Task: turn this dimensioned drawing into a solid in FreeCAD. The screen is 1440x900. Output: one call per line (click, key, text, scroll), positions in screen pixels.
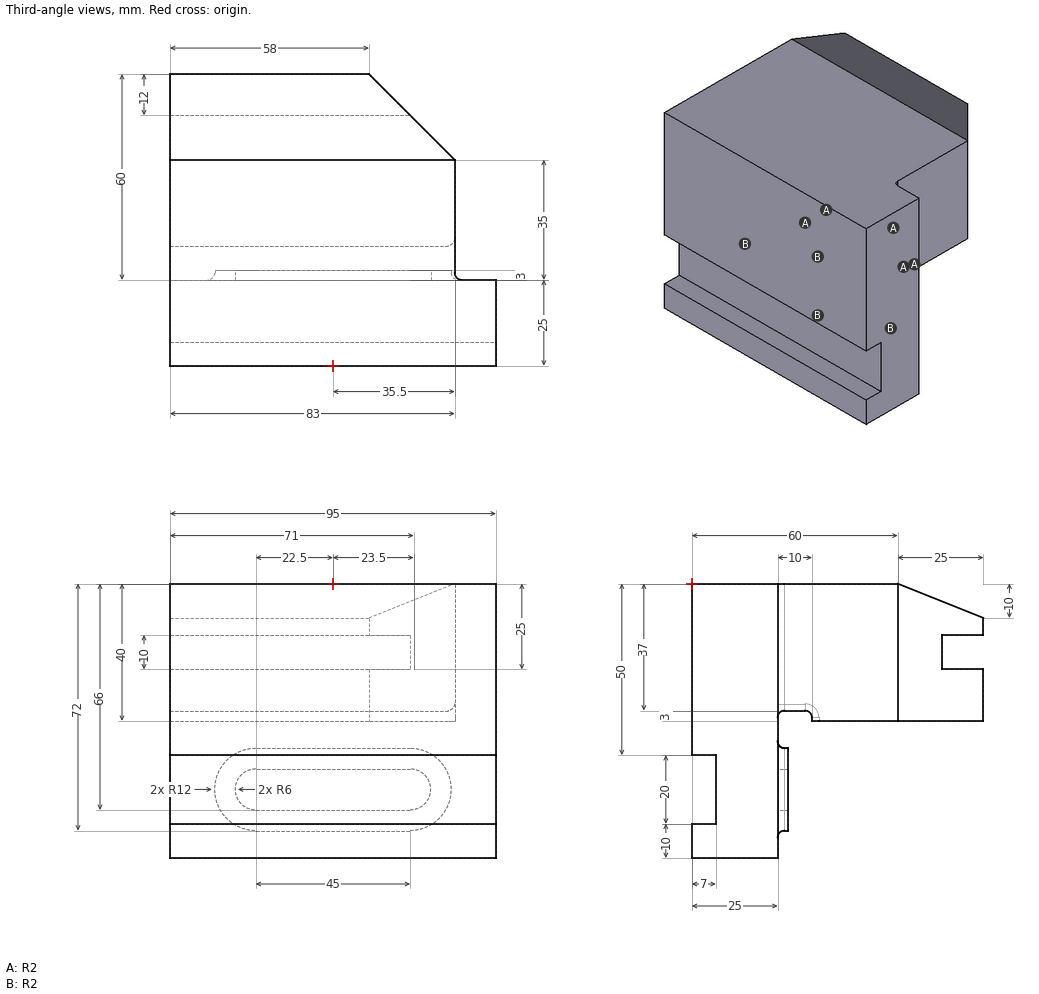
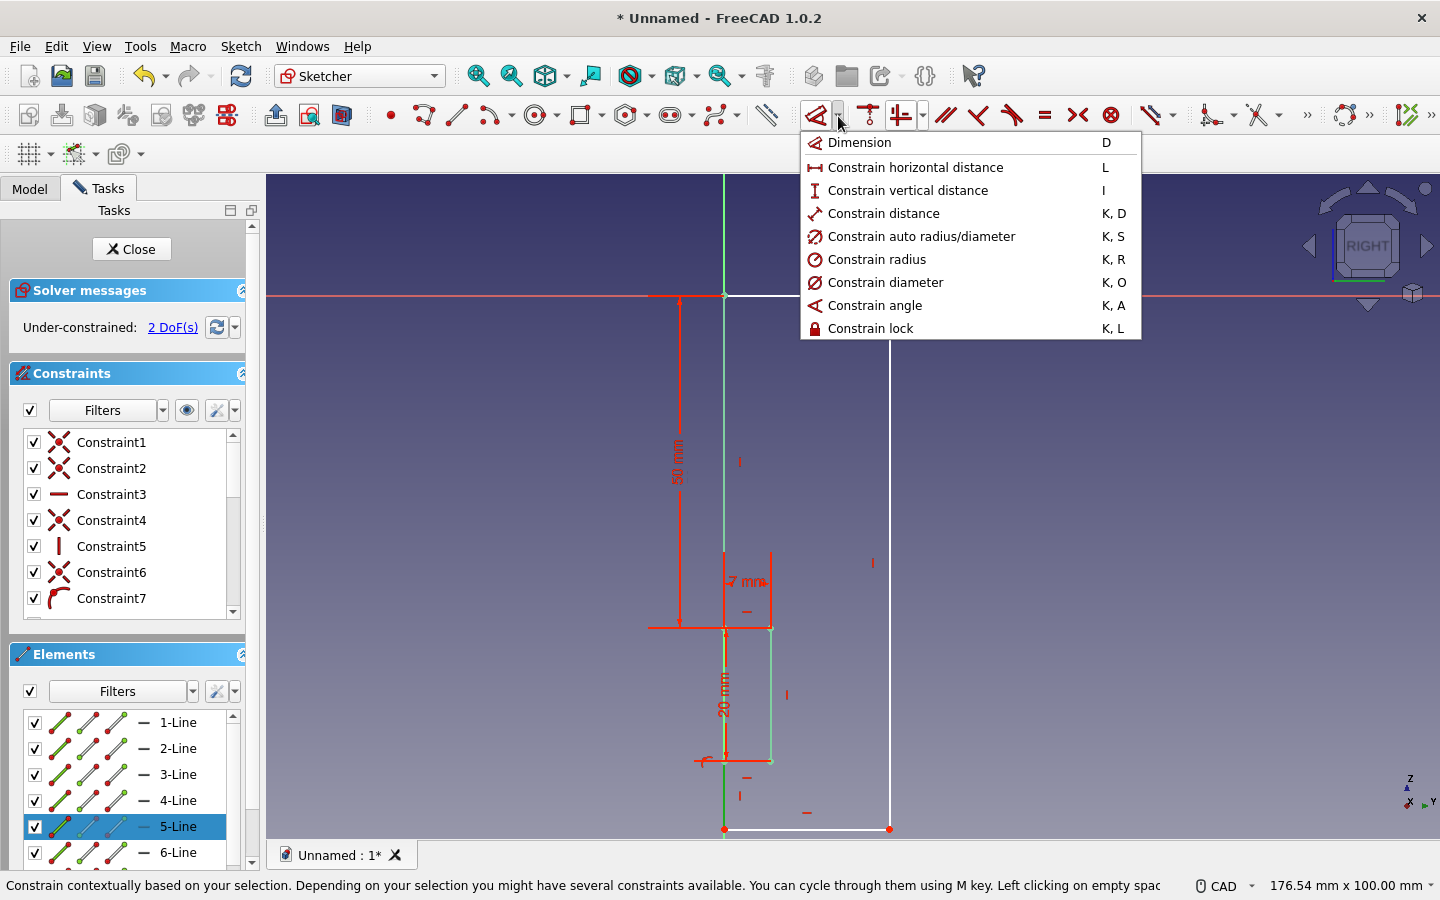
click(971, 190)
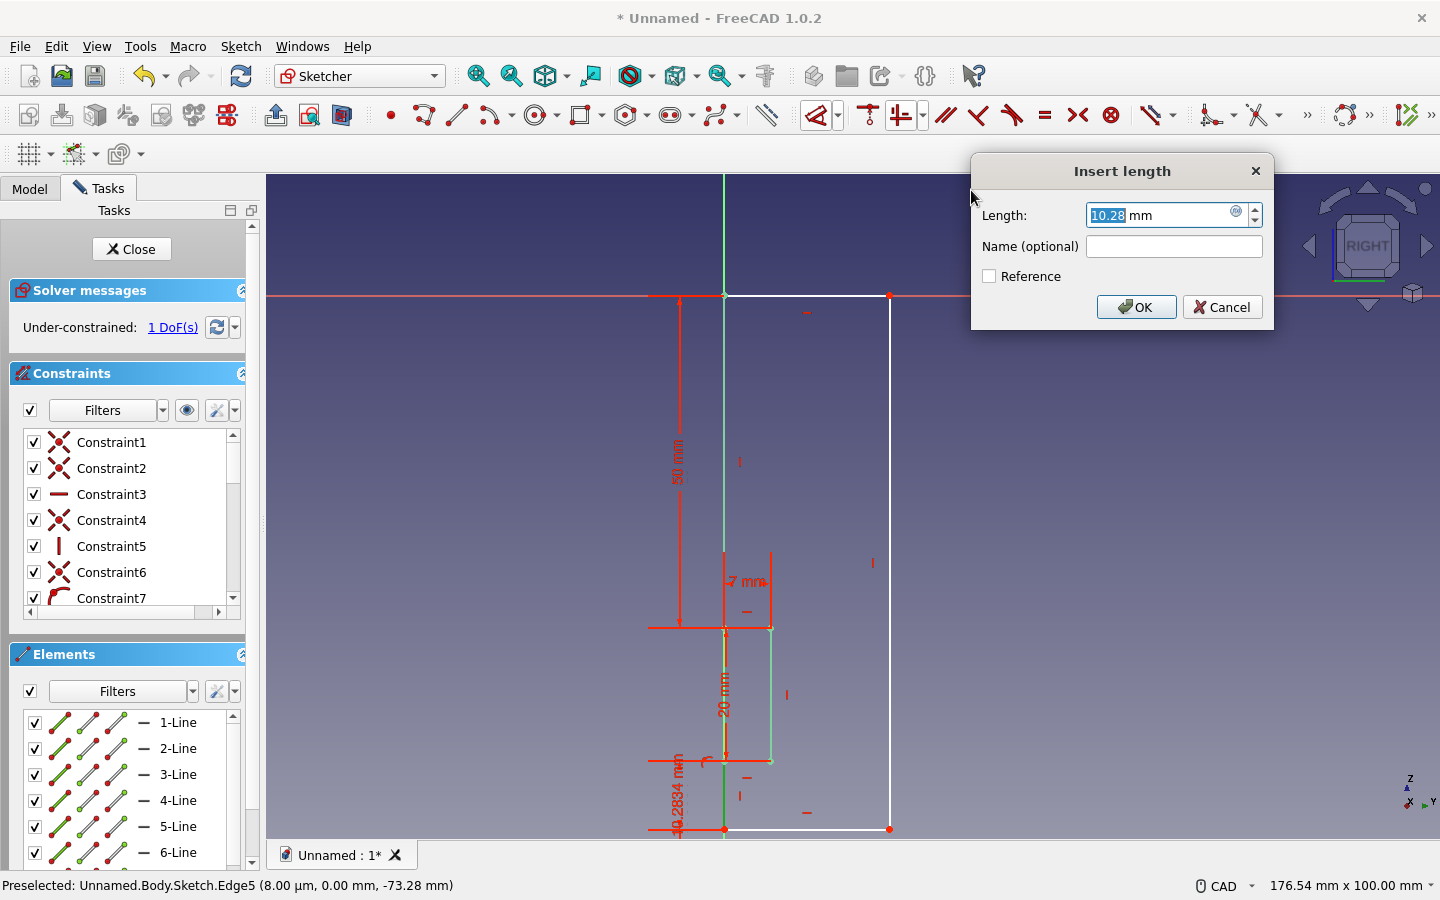
text(10)
key(Return)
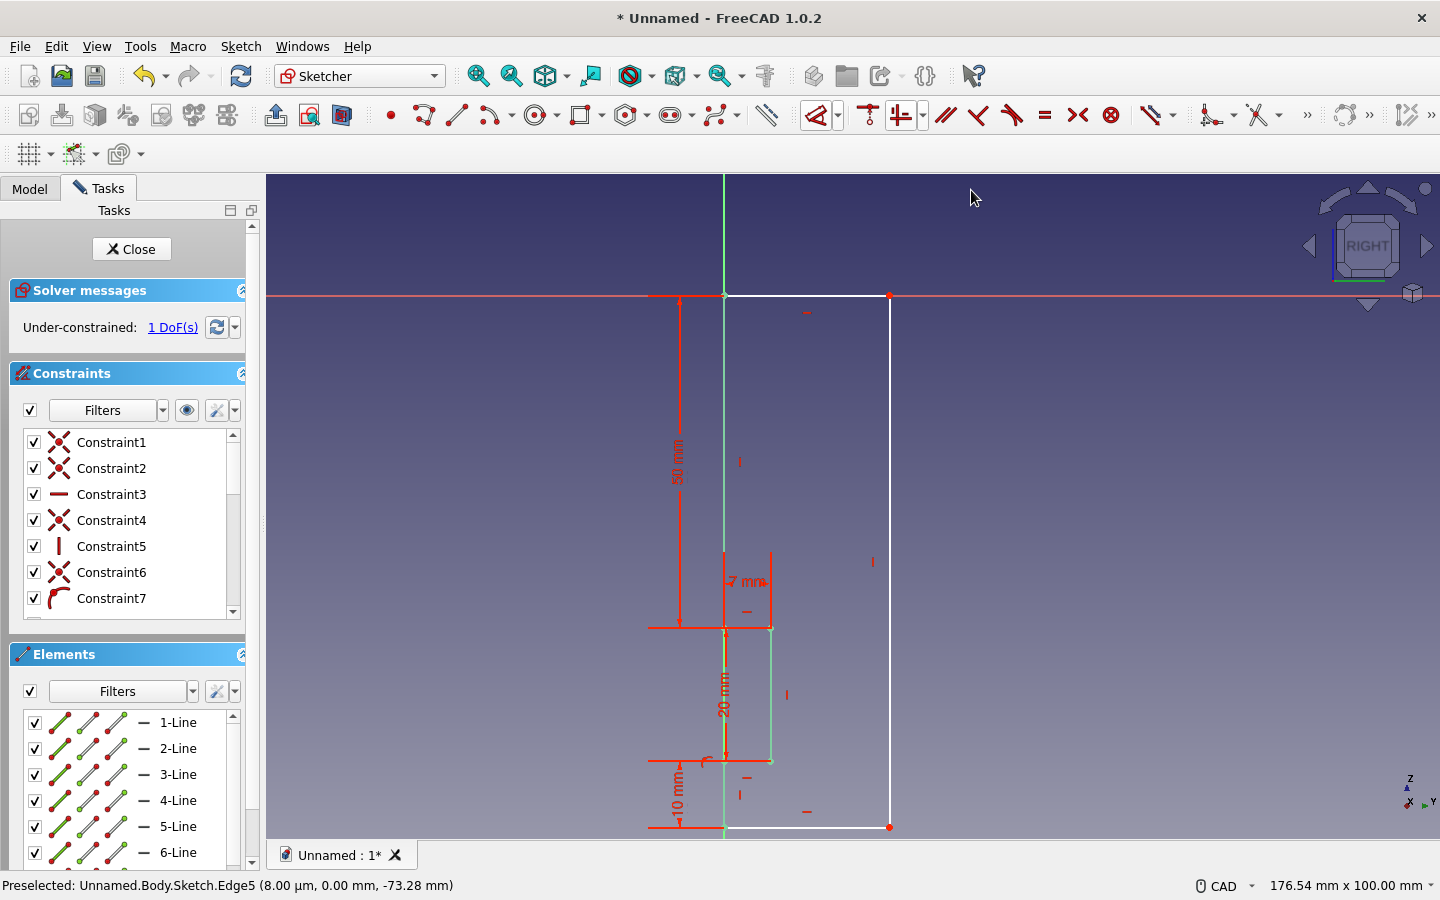
scroll(682, 257, down, 1)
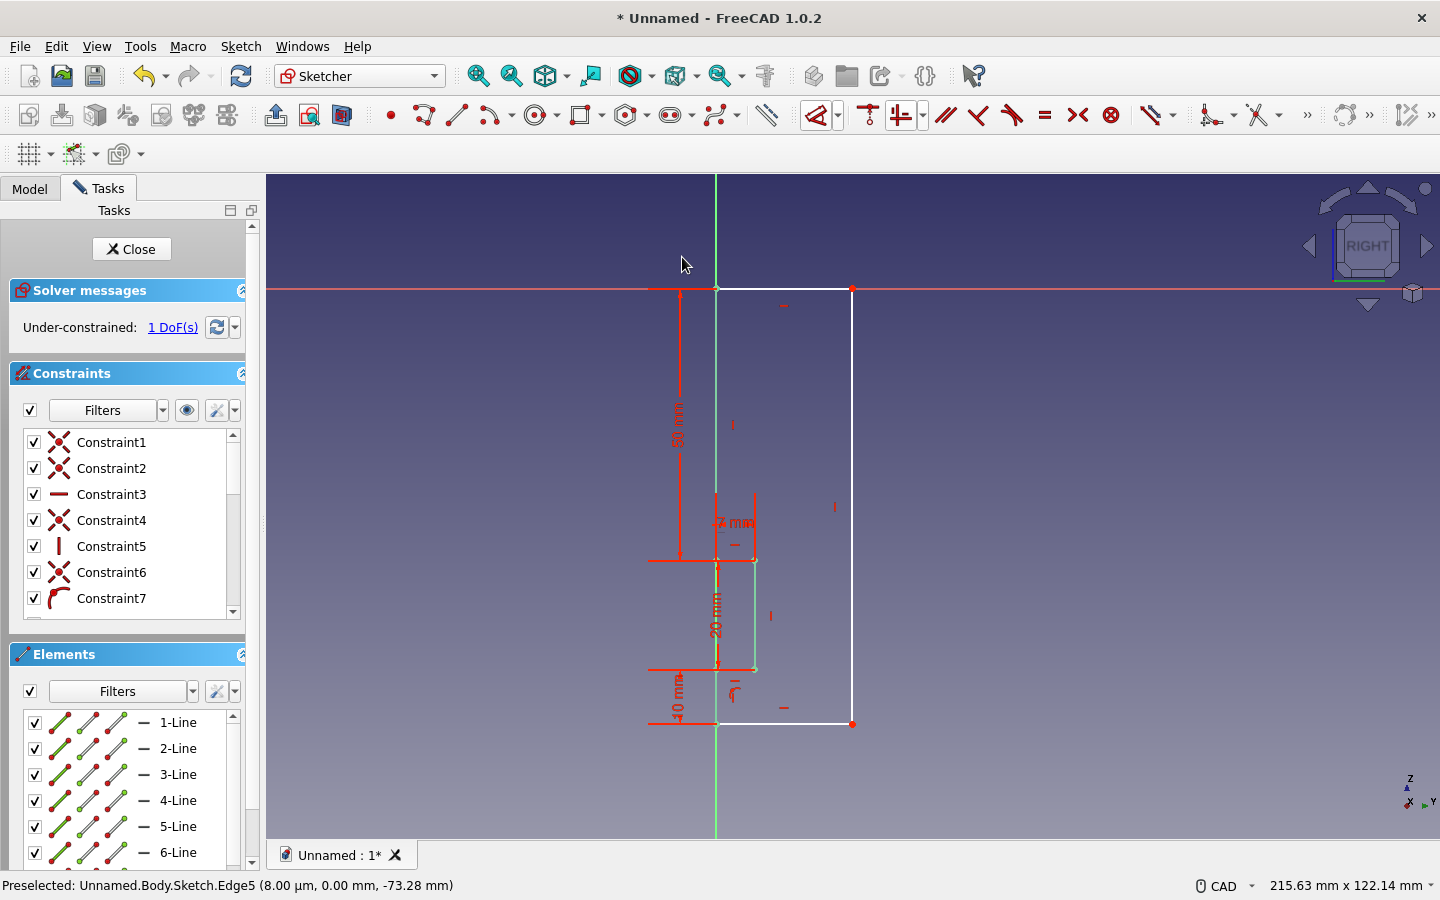
click(757, 724)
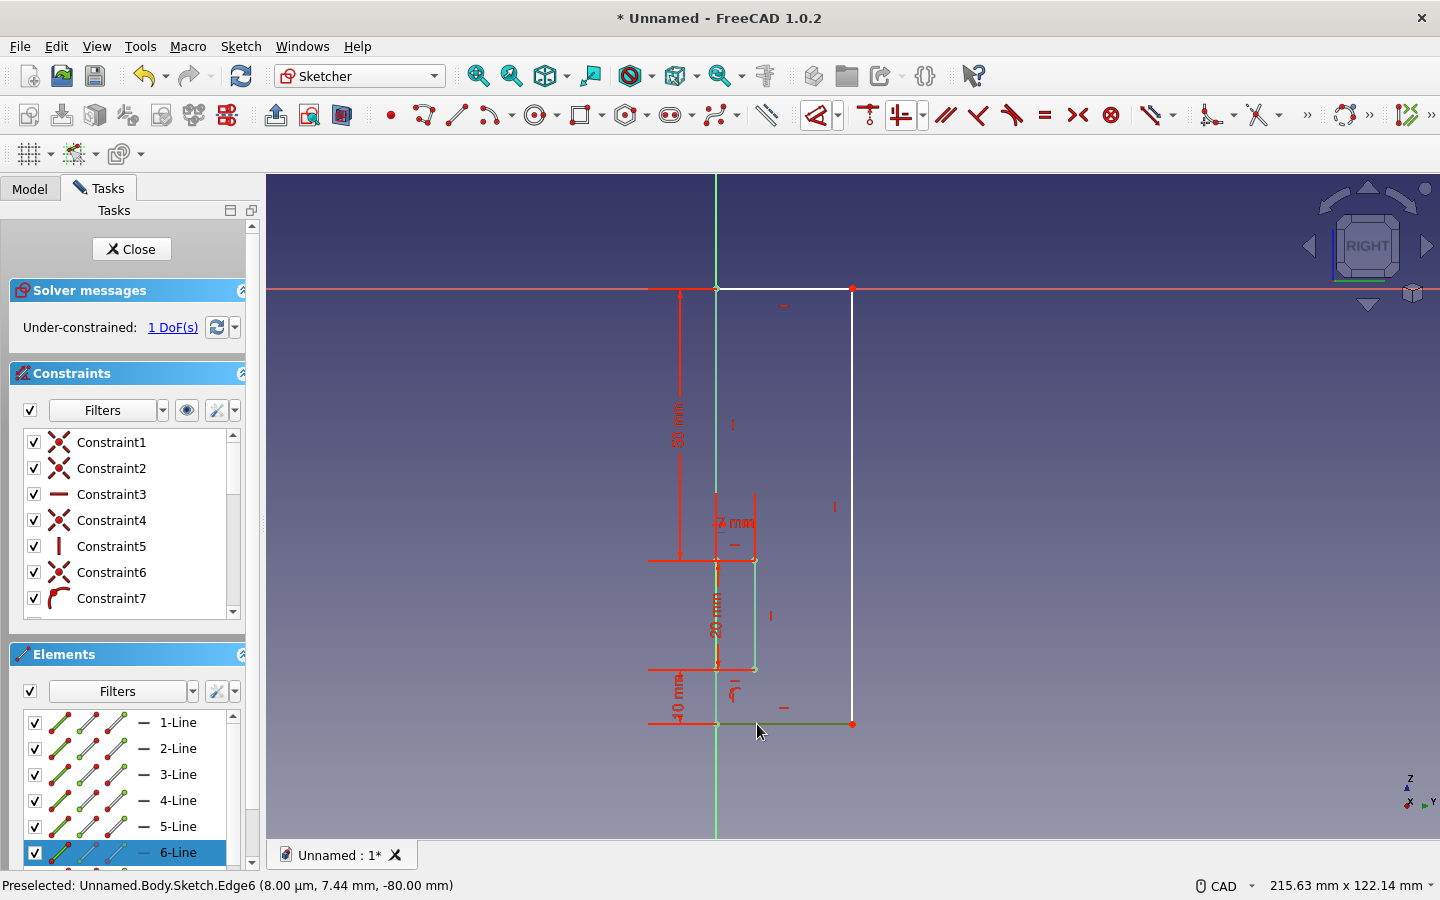
click(838, 116)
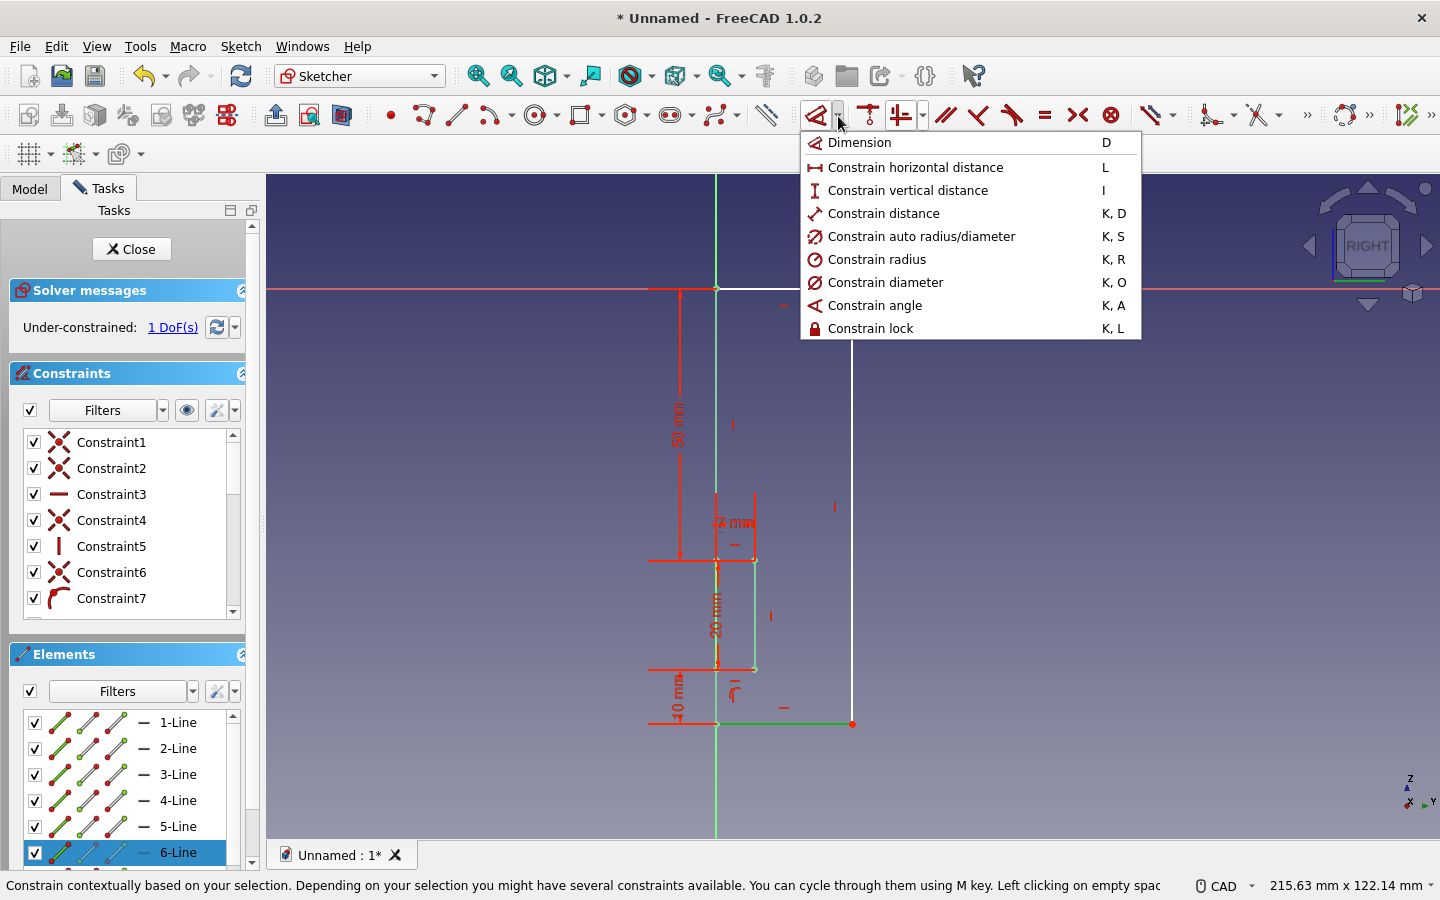
click(971, 168)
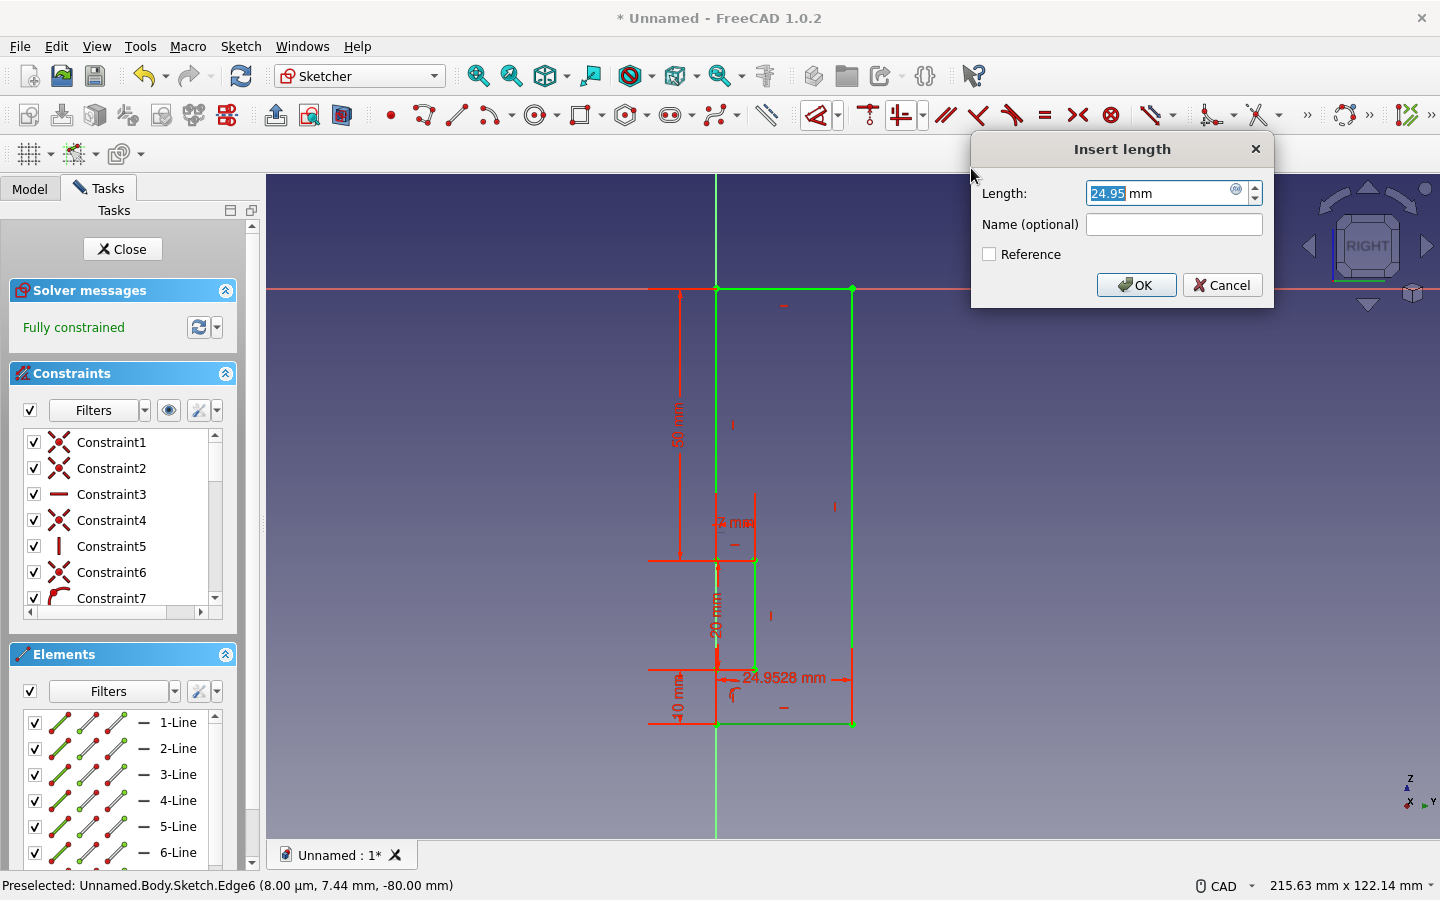
text(25)
key(Return)